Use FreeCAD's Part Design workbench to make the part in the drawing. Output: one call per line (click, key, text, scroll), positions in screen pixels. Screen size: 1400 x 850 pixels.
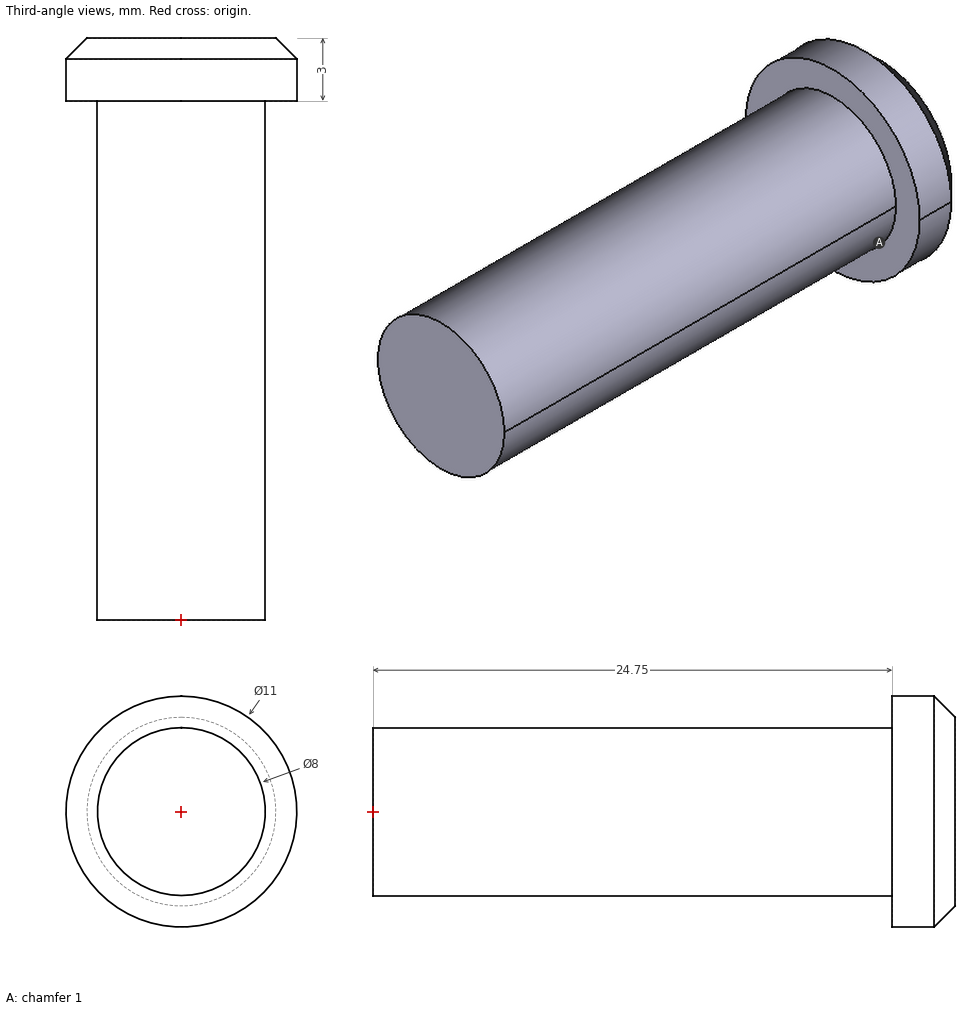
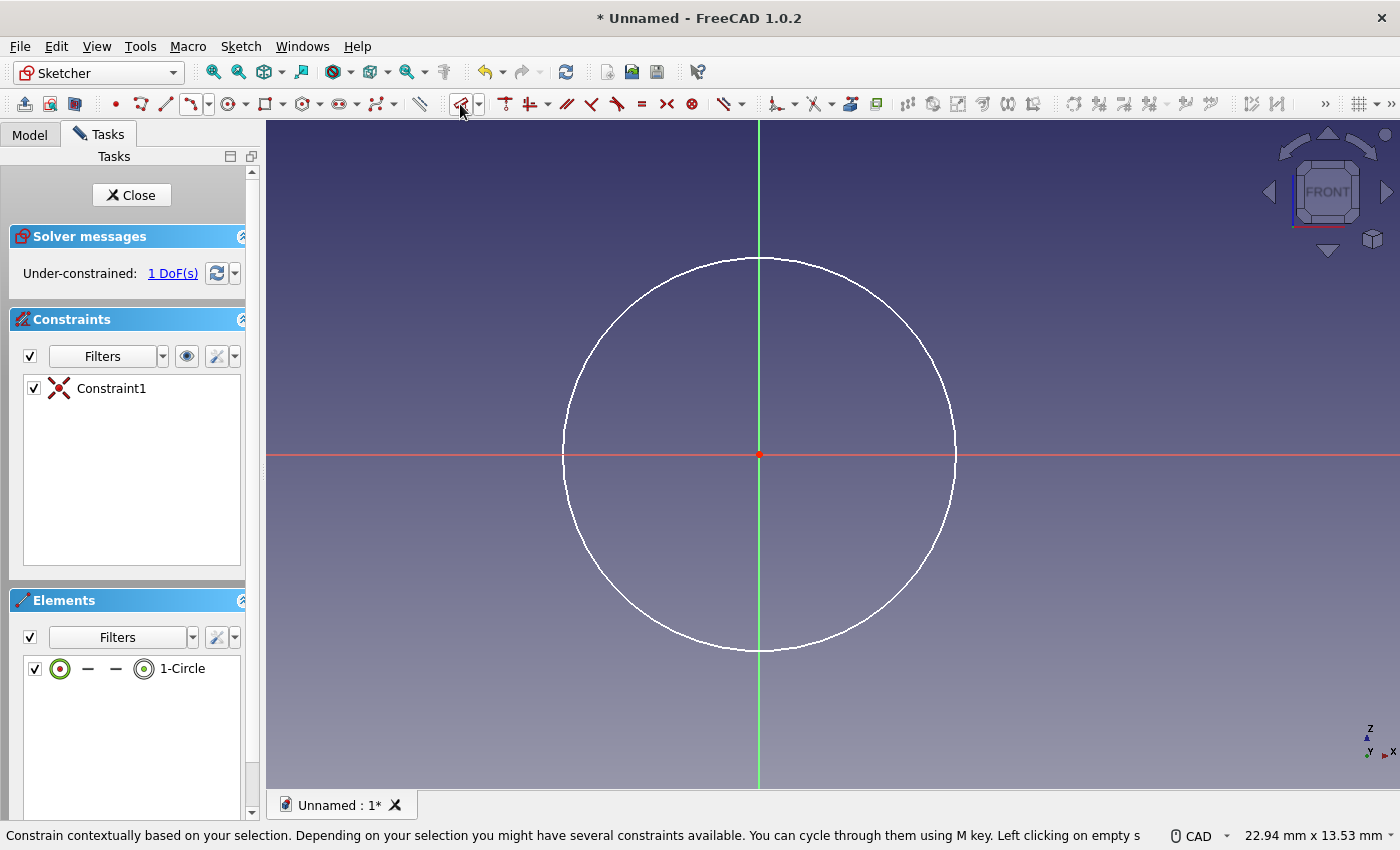
click(898, 315)
click(921, 292)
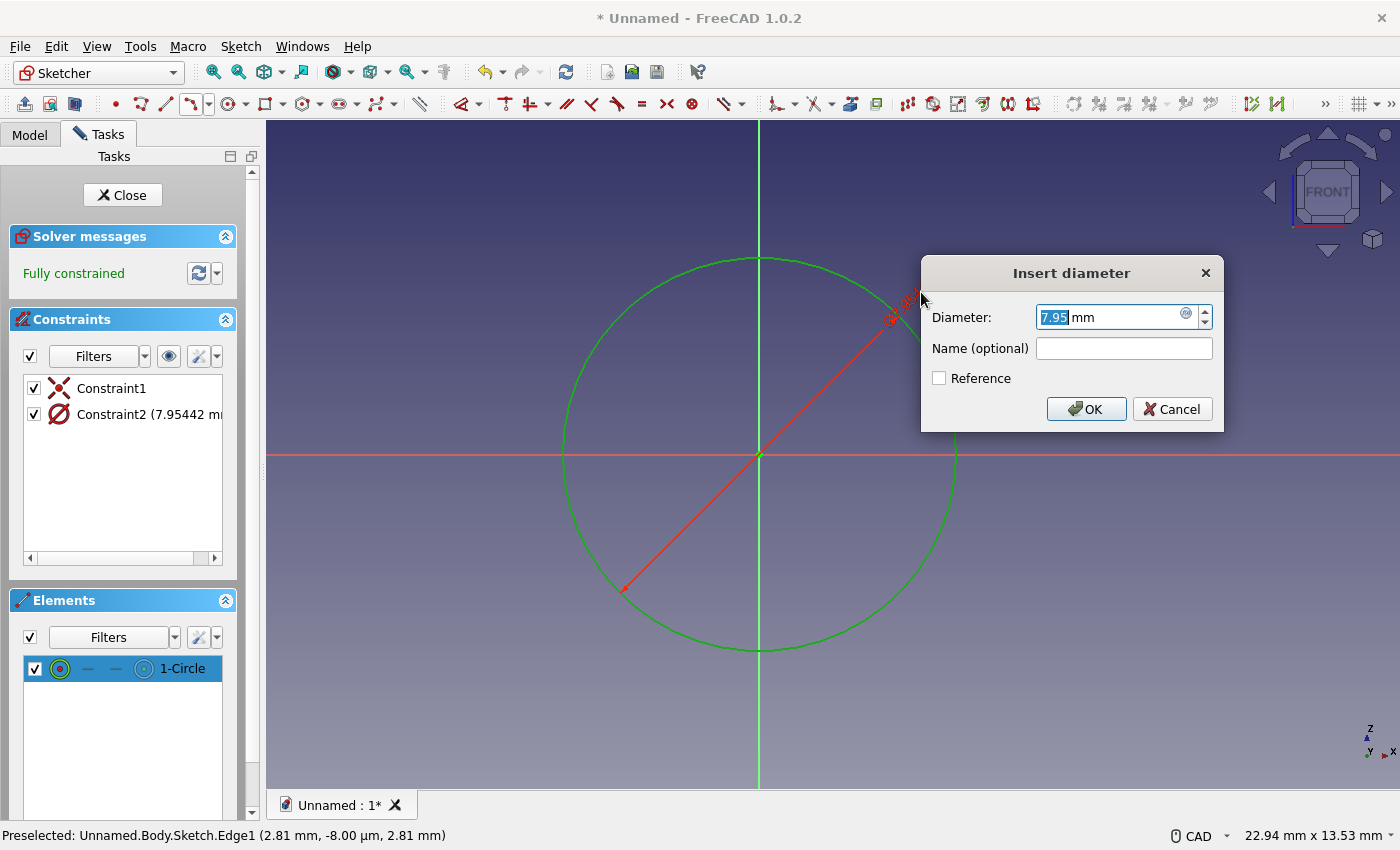
text(8)
key(Return)
key(Escape)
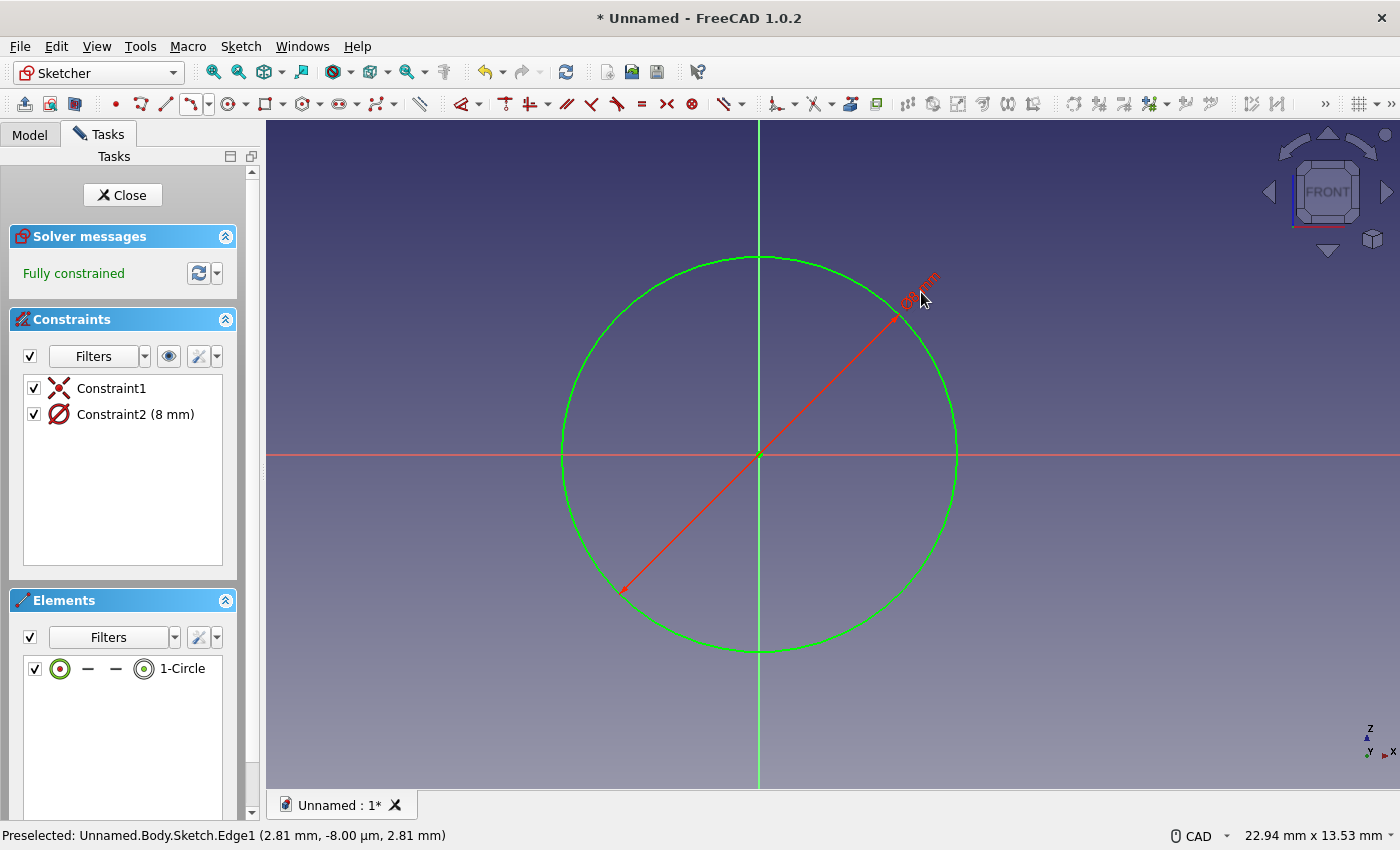
click(123, 195)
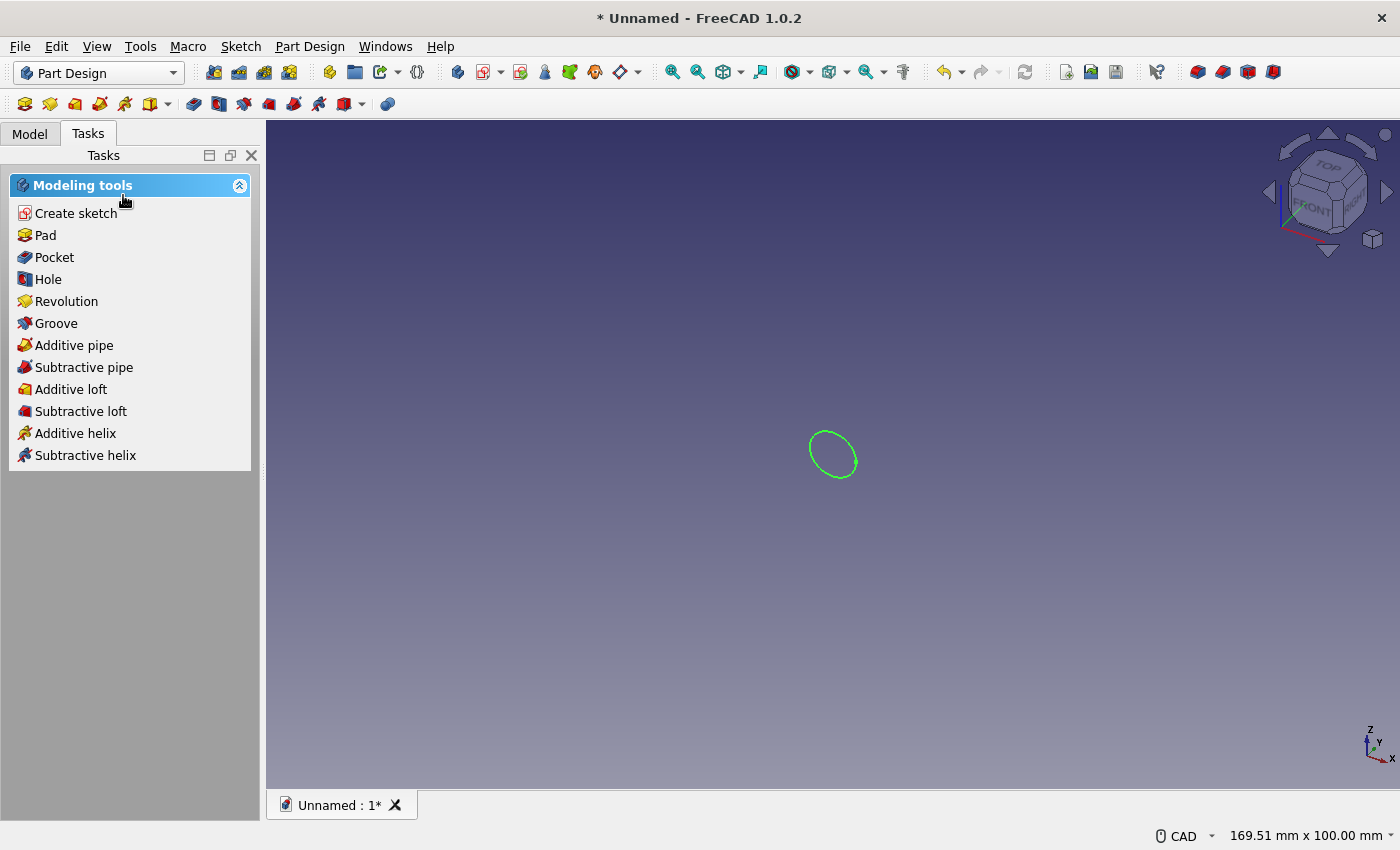
click(25, 104)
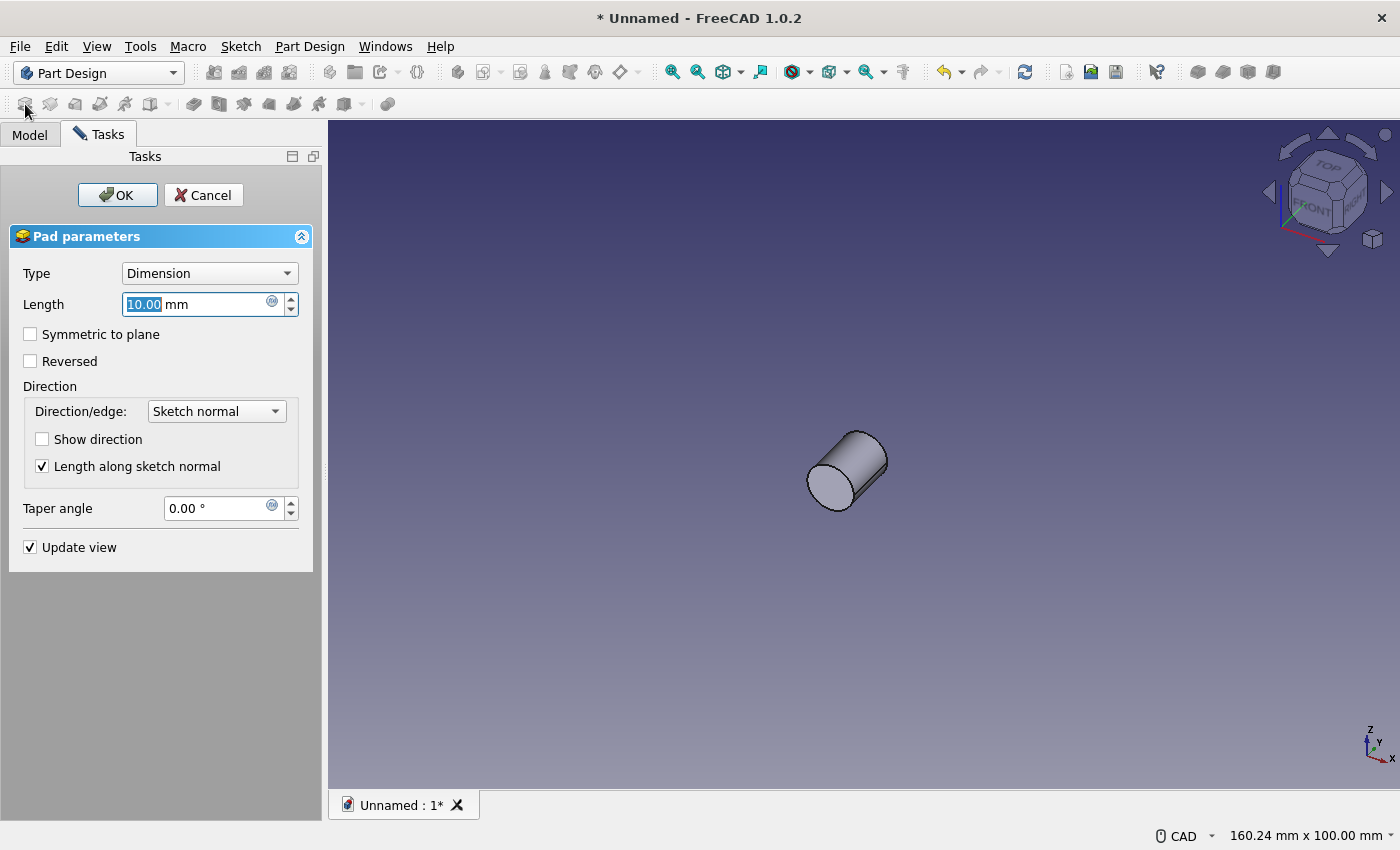
text(24.75)
key(Tab)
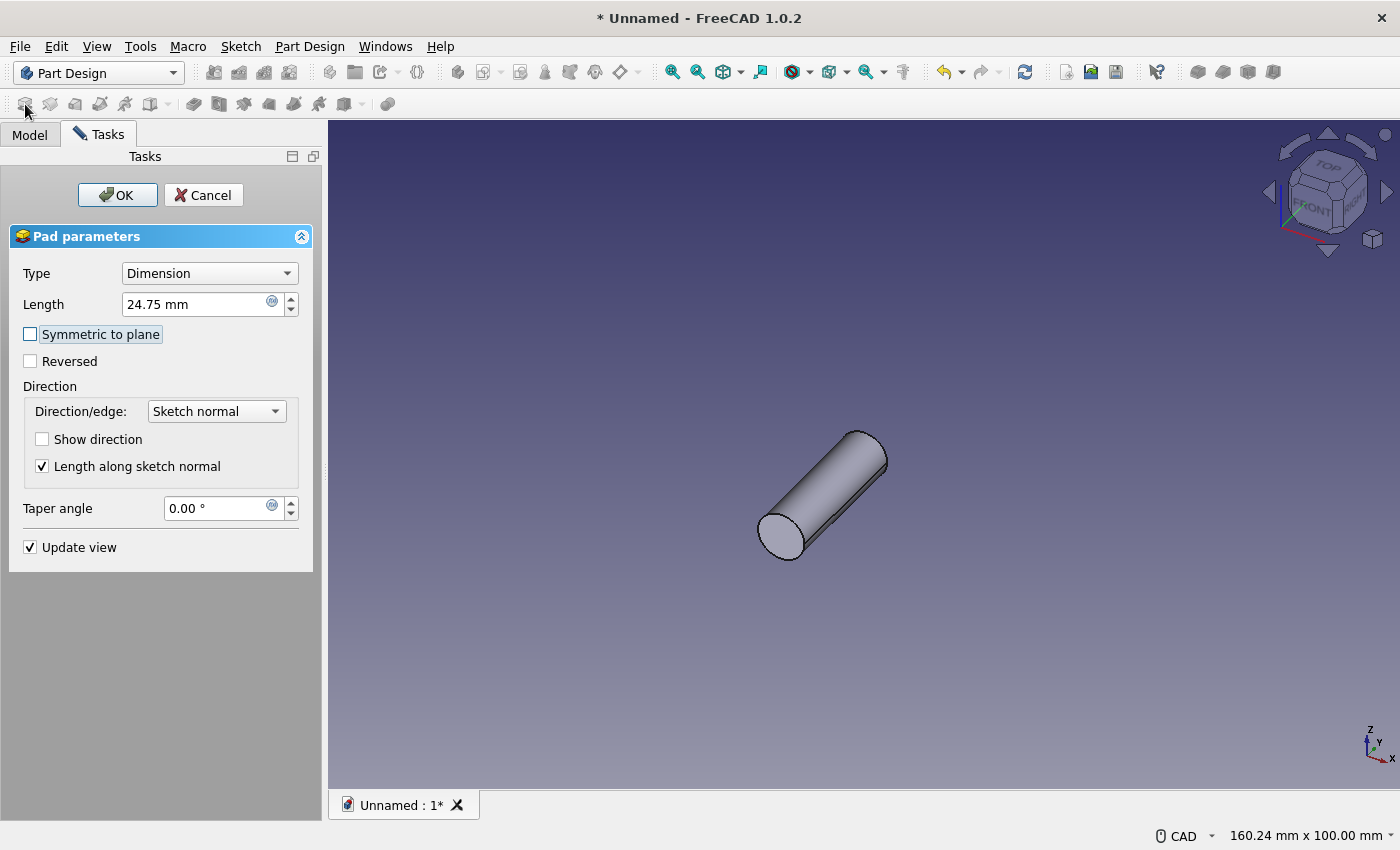
click(31, 361)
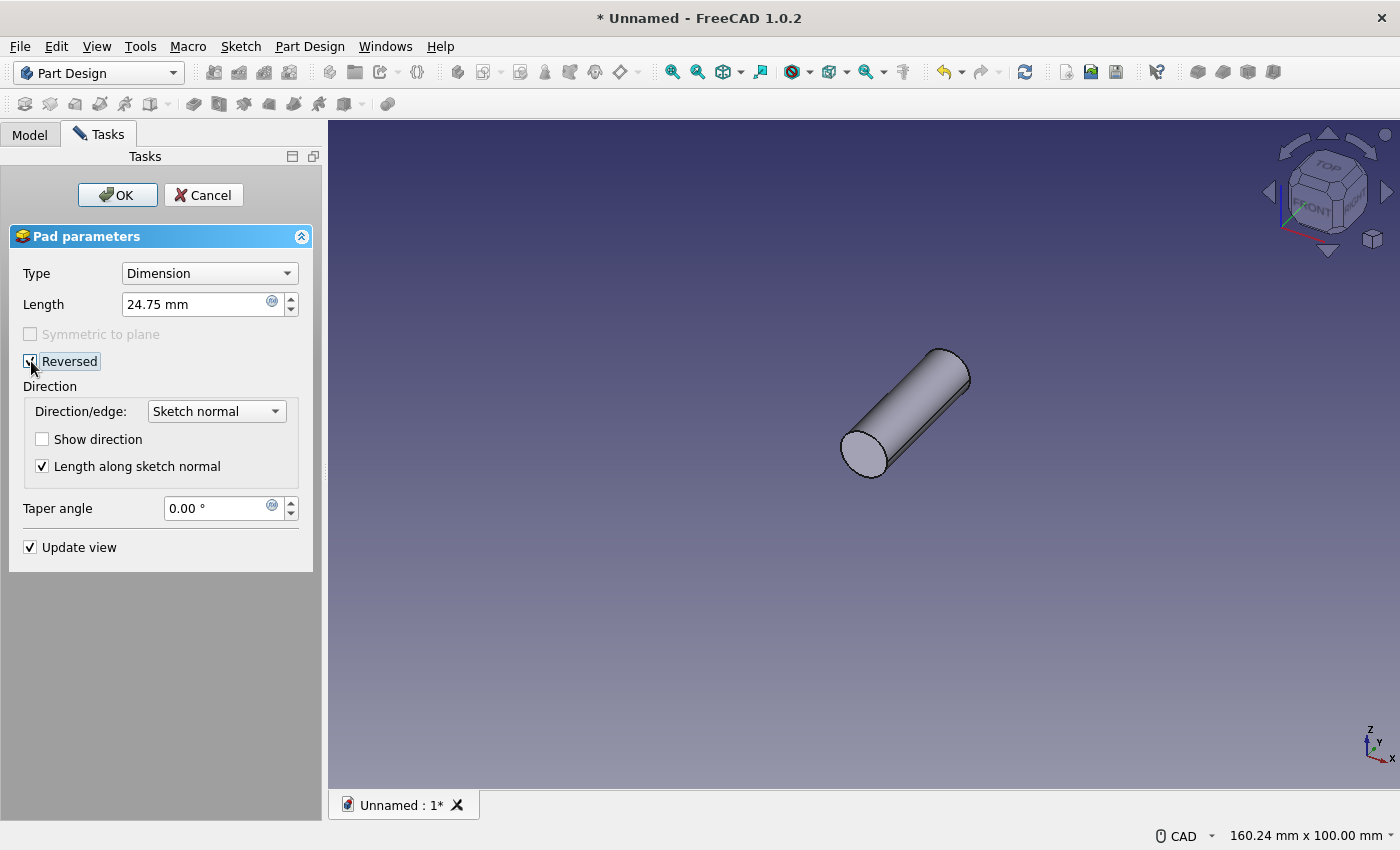
click(118, 195)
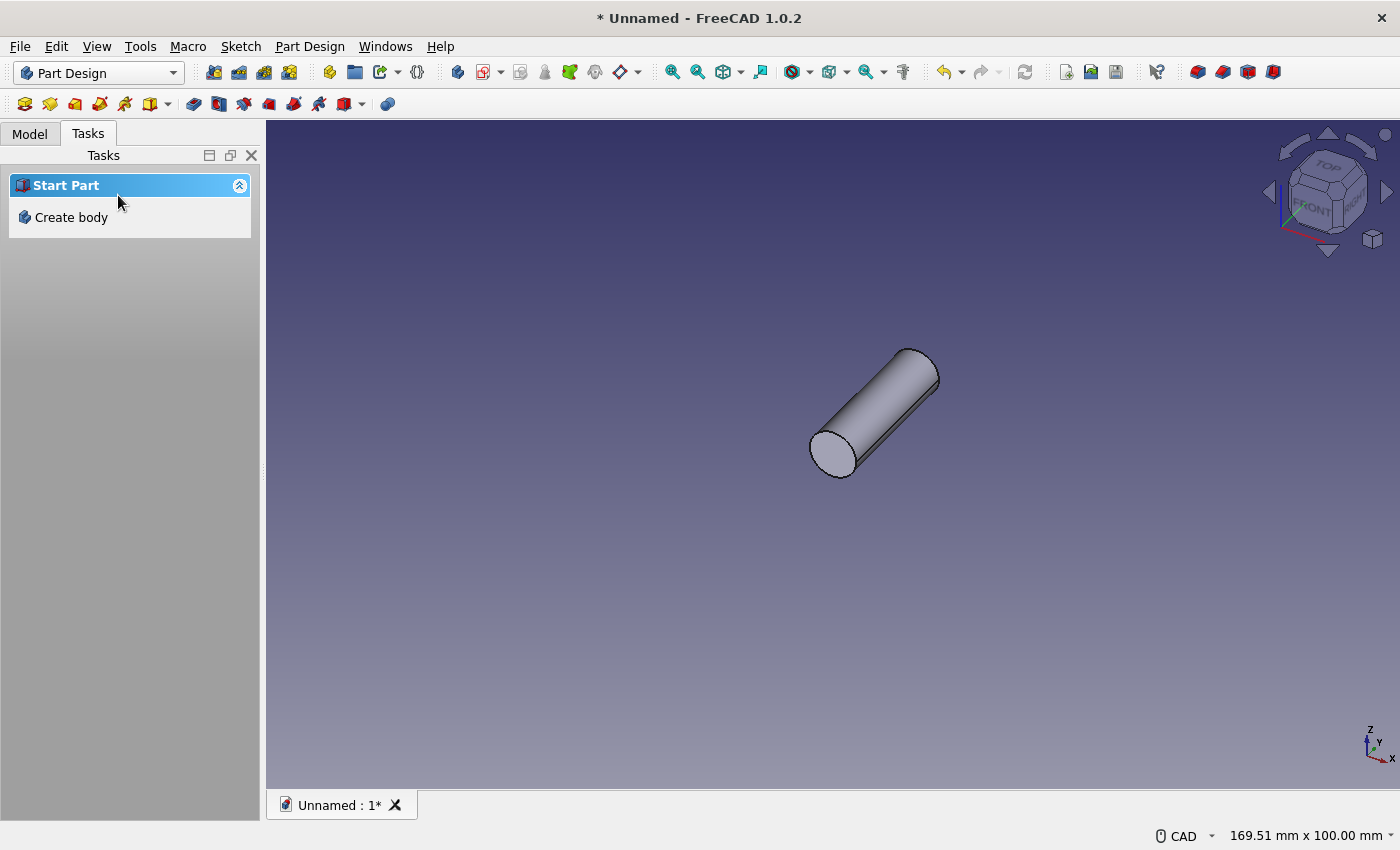
click(673, 72)